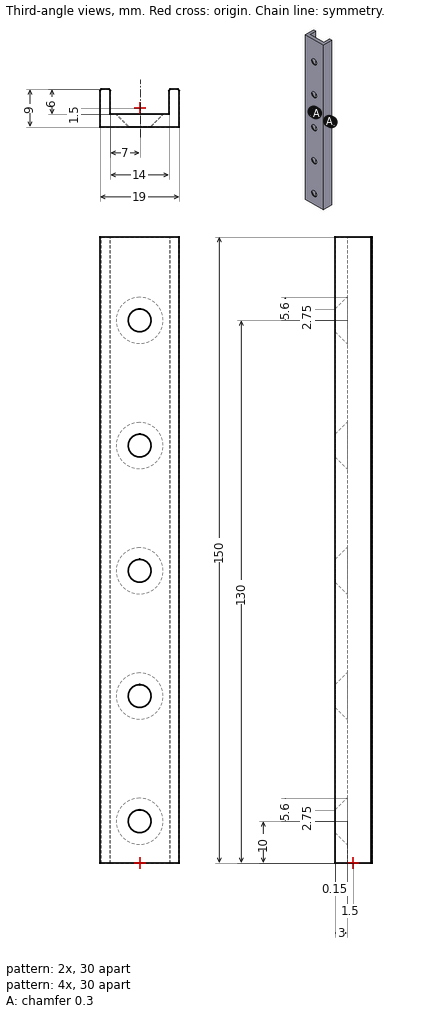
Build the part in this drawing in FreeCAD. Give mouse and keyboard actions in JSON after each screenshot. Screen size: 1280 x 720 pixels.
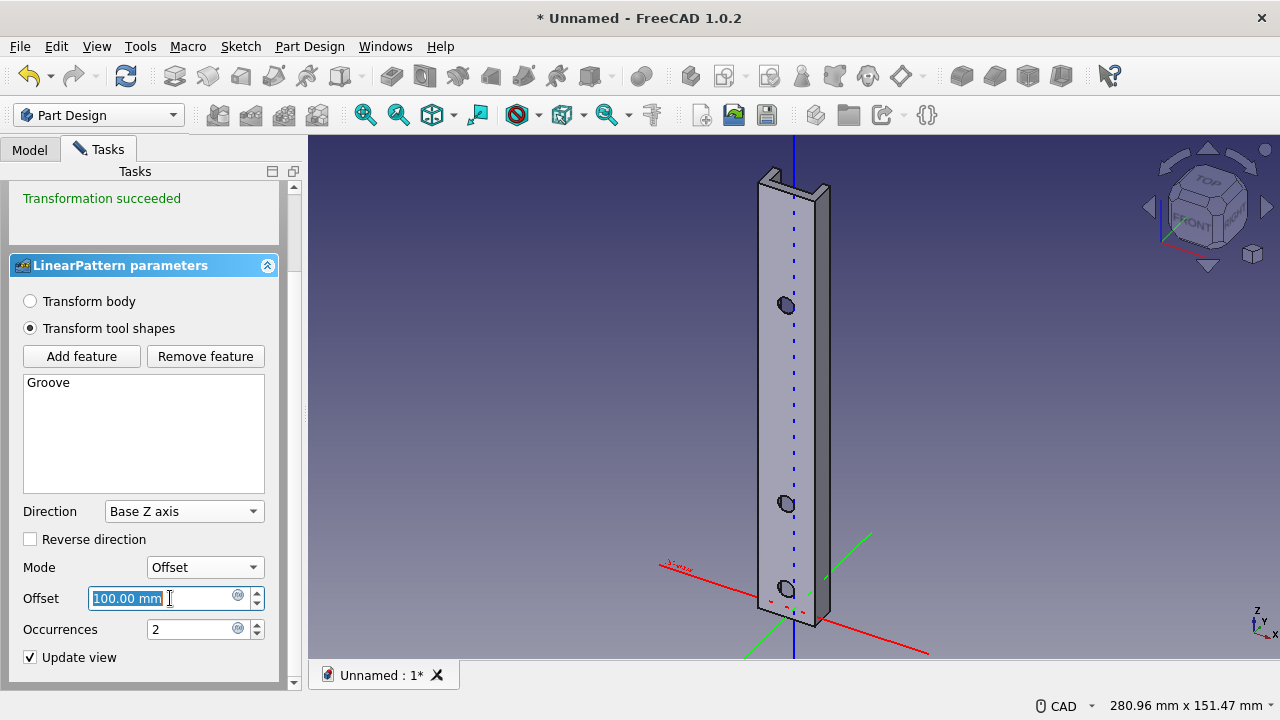
{"action": "type", "text": "30"}
{"action": "key", "text": "Tab"}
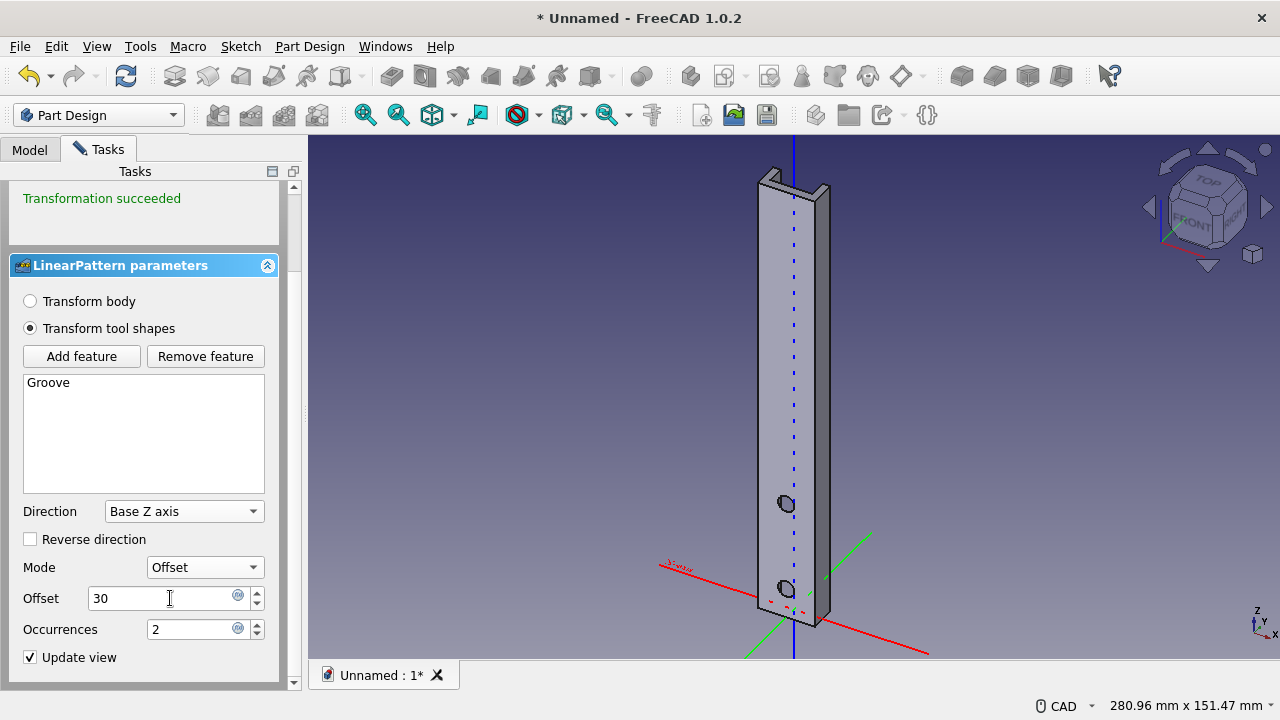
{"action": "triple_click", "coordinate": [199, 630]}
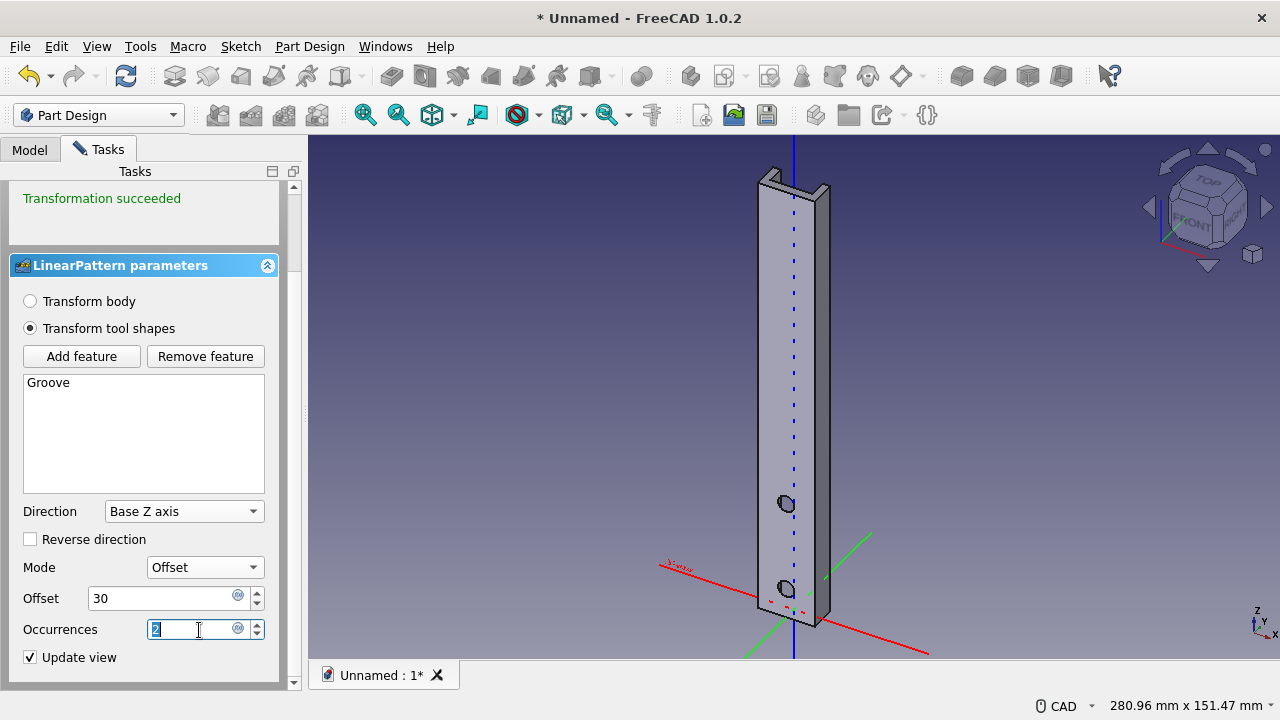
{"action": "type", "text": "4"}
{"action": "key", "text": "Tab"}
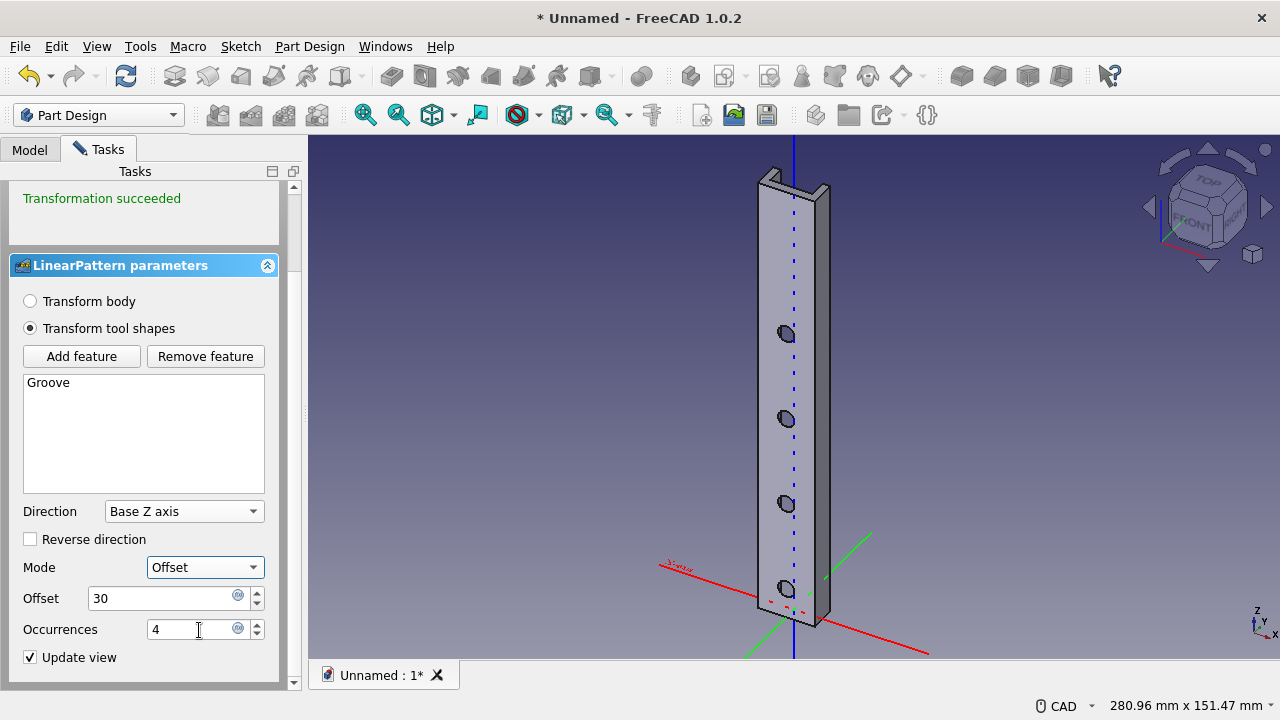
{"action": "scroll", "coordinate": [294, 436], "scroll_direction": "up", "scroll_amount": 3}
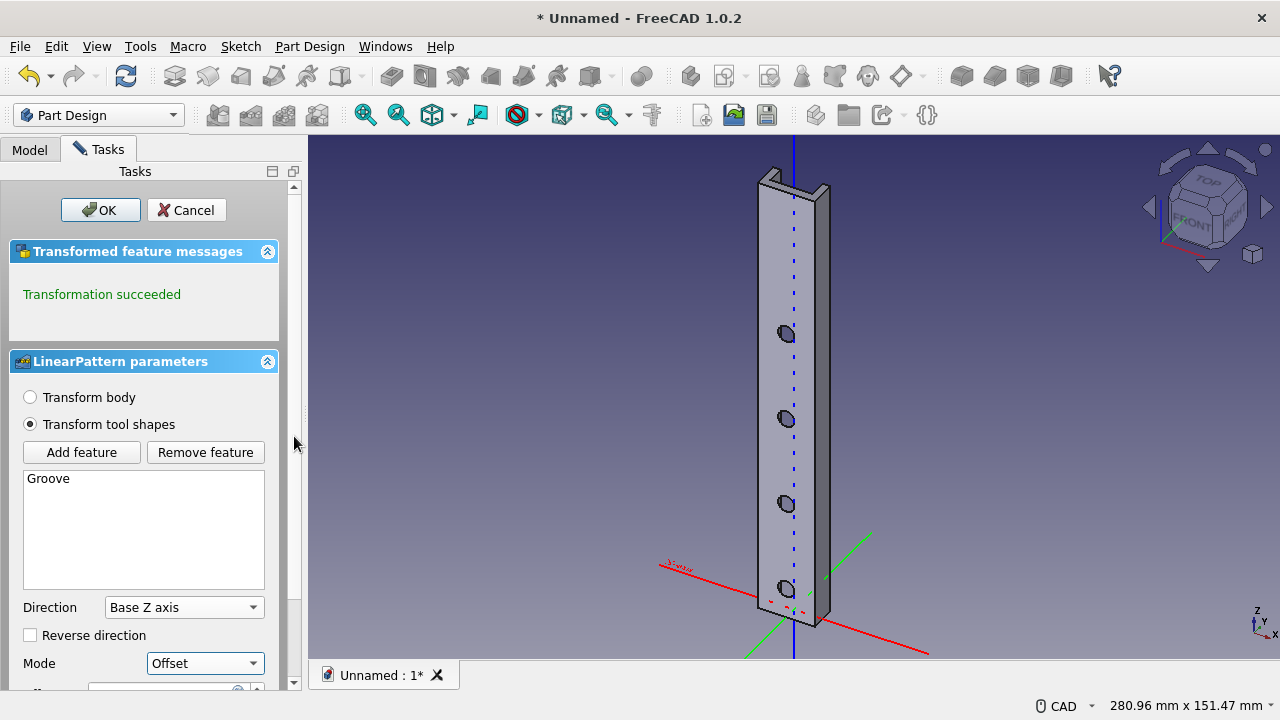
{"action": "left_click", "coordinate": [101, 210]}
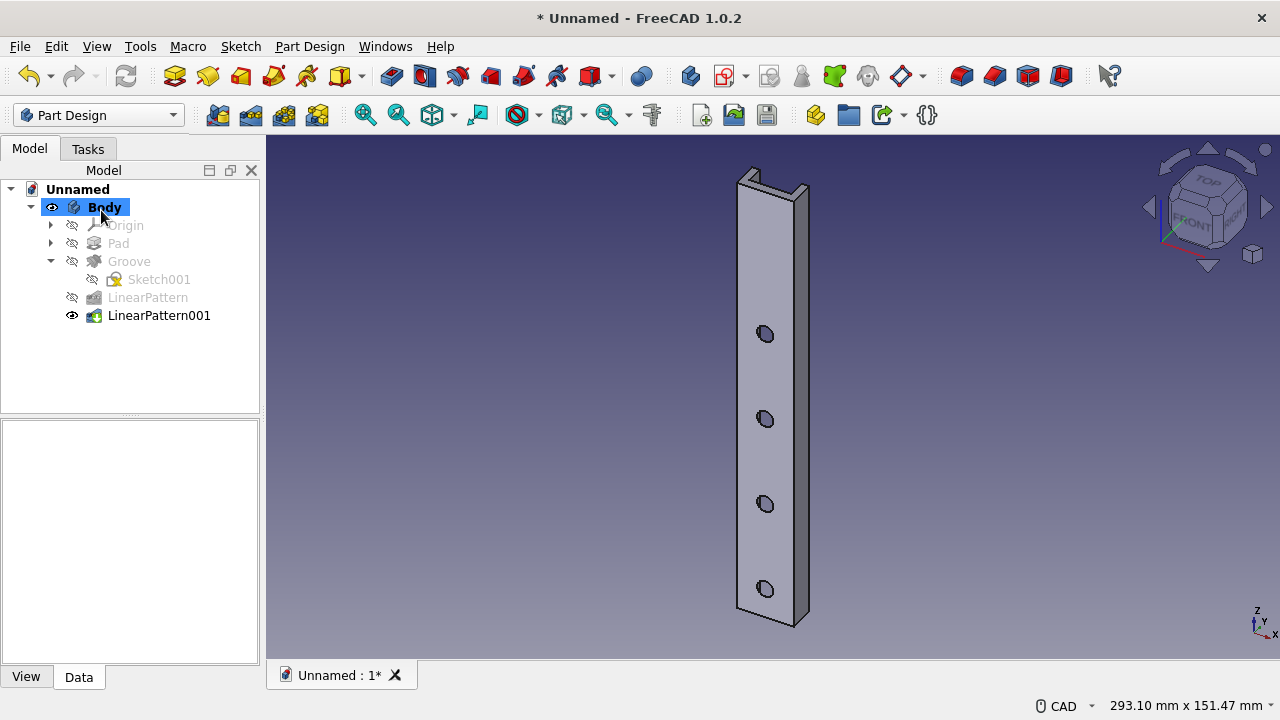
{"action": "left_click", "coordinate": [724, 76]}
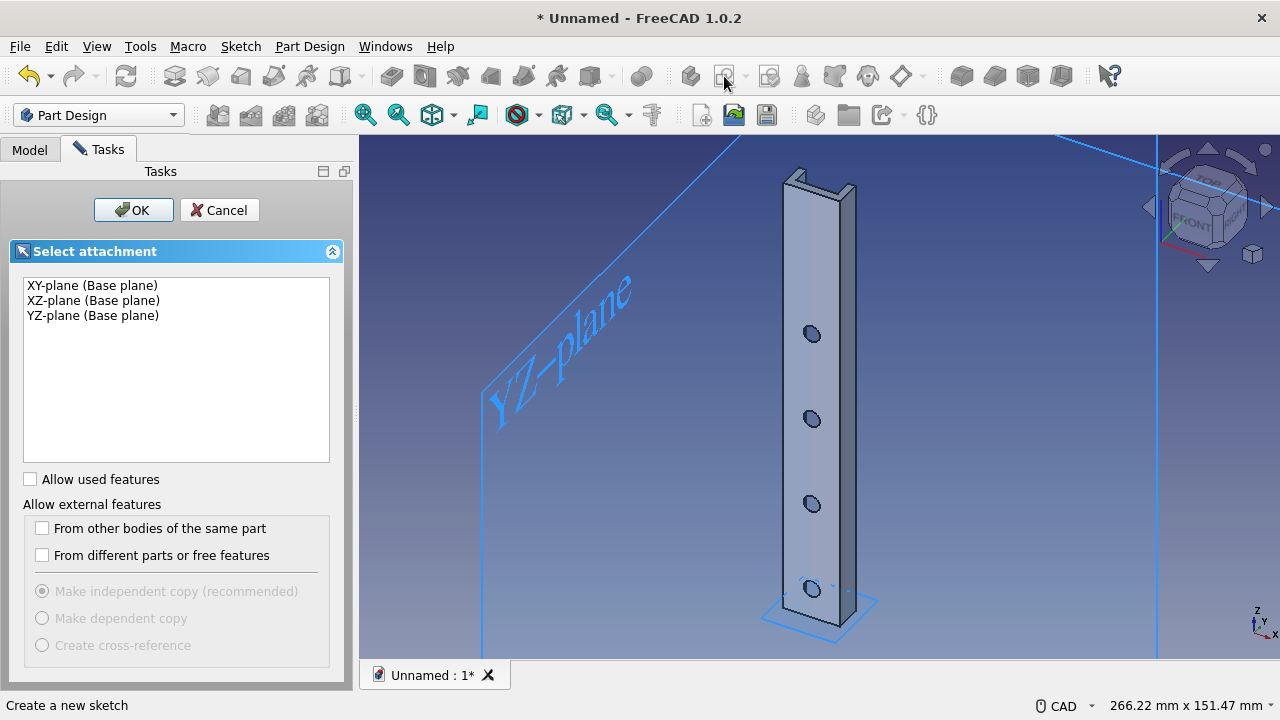
{"action": "left_click", "coordinate": [84, 316]}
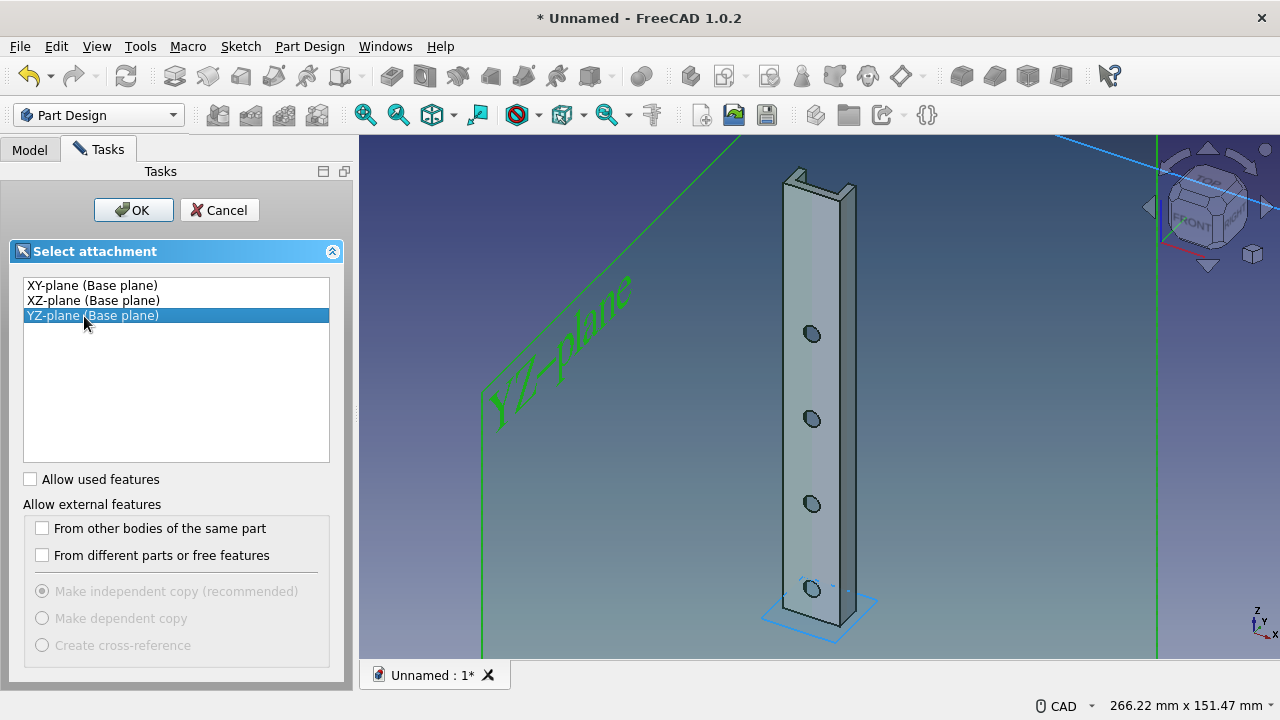
{"action": "left_click", "coordinate": [134, 210]}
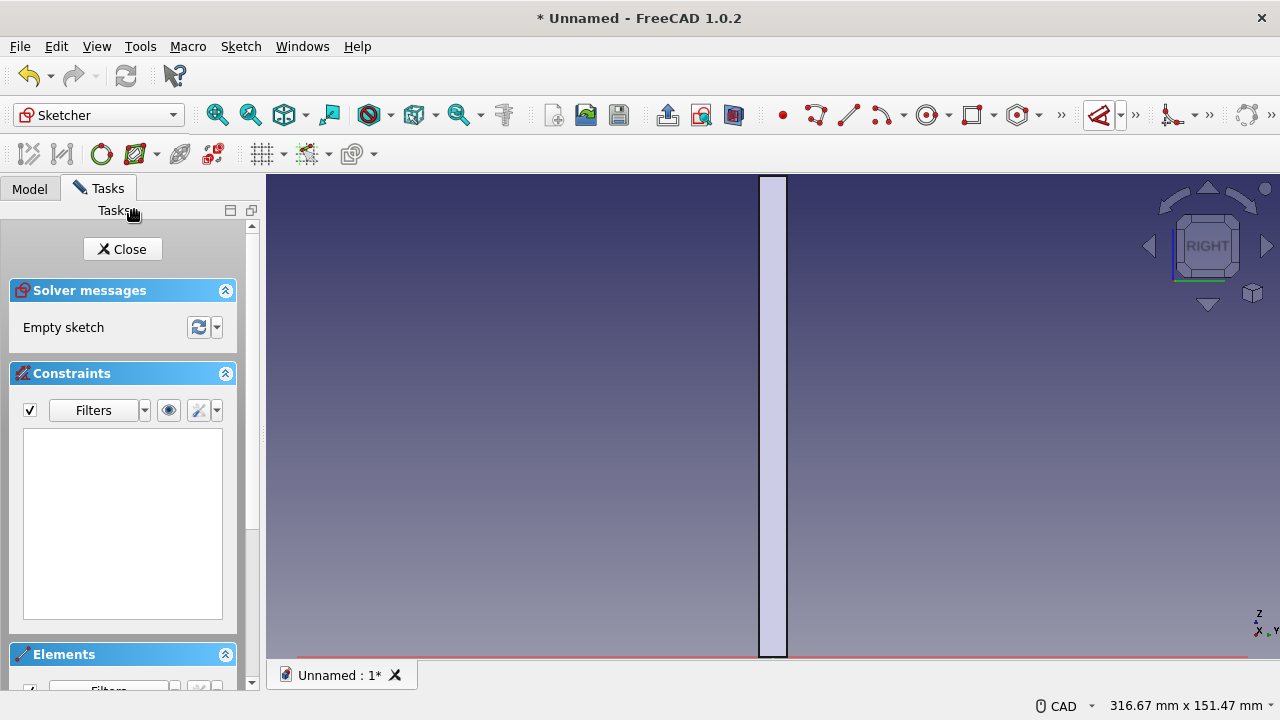
{"action": "left_click", "coordinate": [734, 116]}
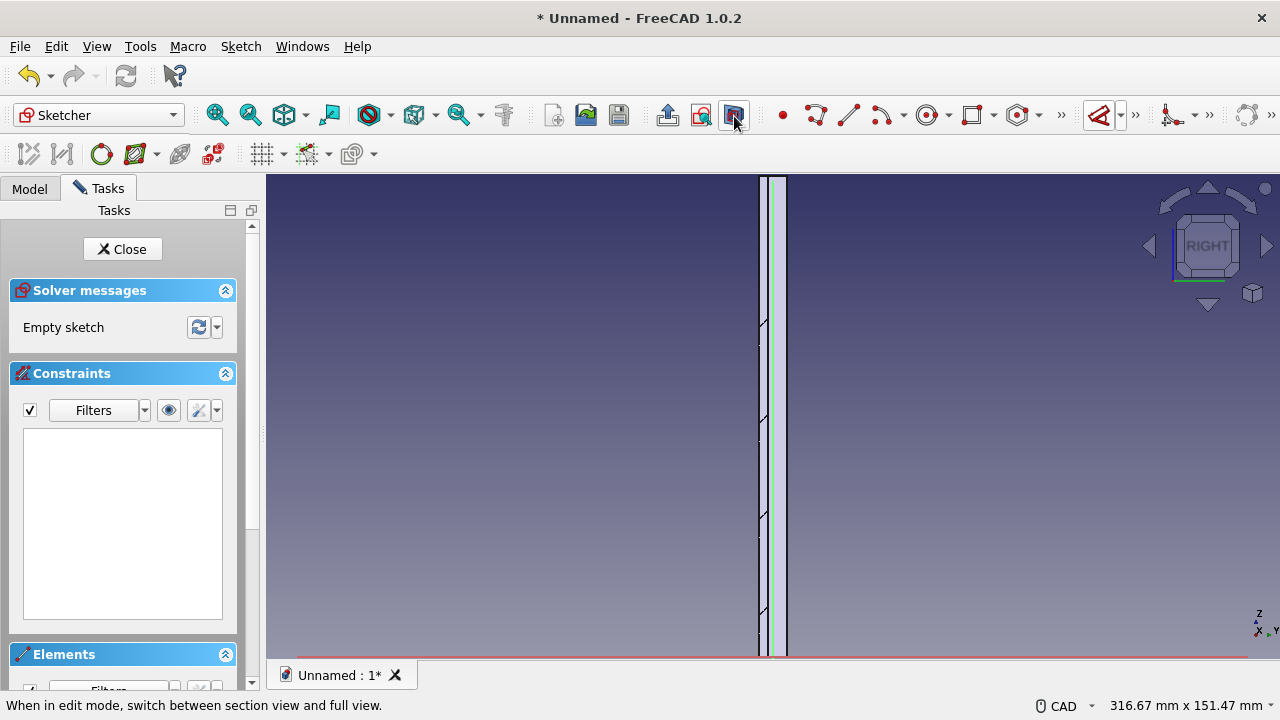
{"action": "scroll", "coordinate": [765, 219], "scroll_direction": "up", "scroll_amount": 14}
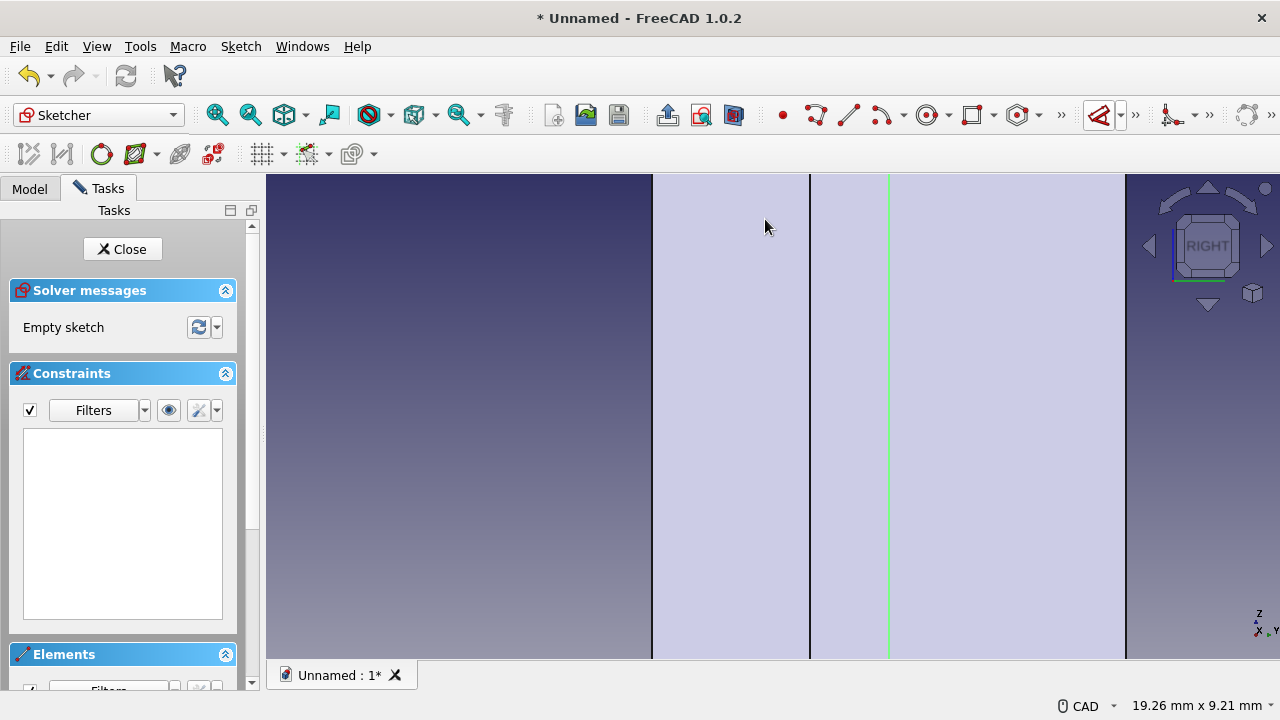
{"action": "left_click", "coordinate": [816, 116]}